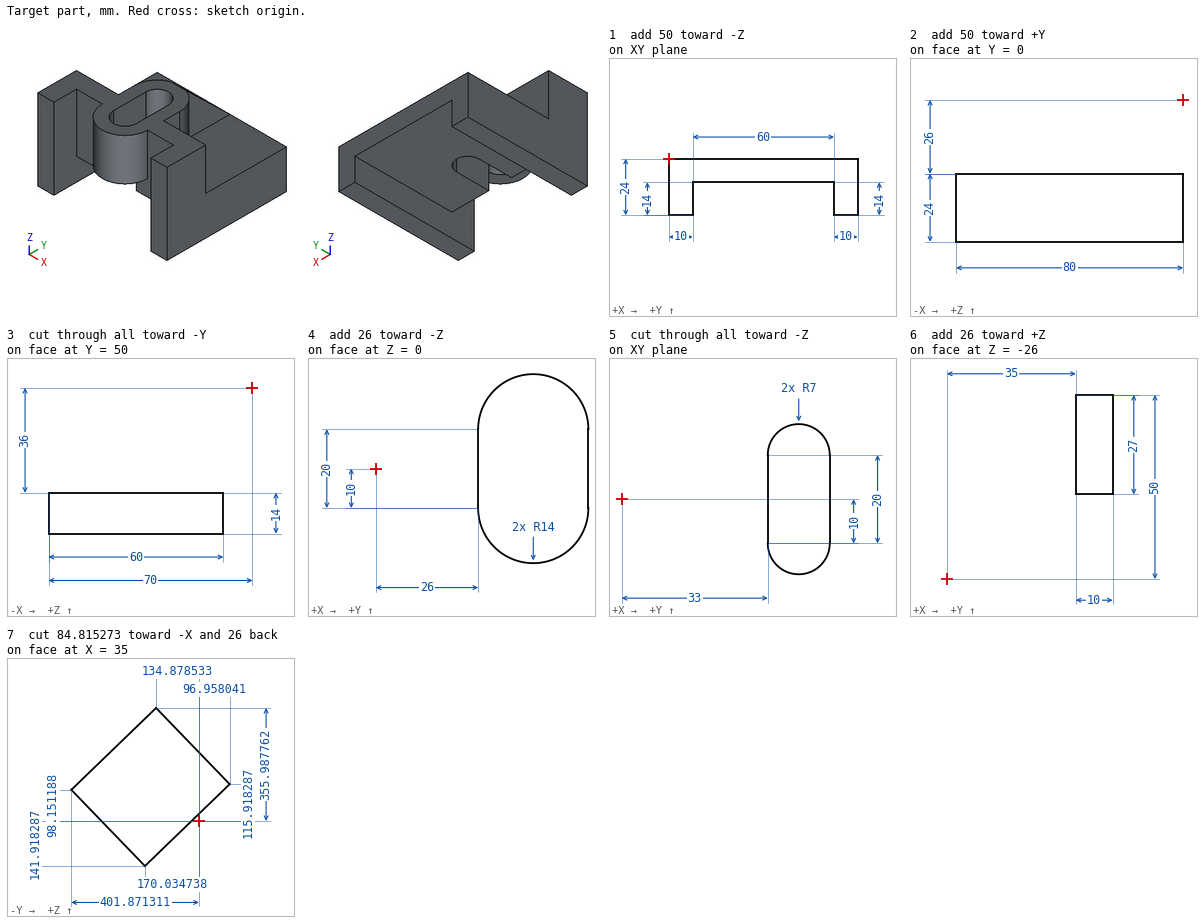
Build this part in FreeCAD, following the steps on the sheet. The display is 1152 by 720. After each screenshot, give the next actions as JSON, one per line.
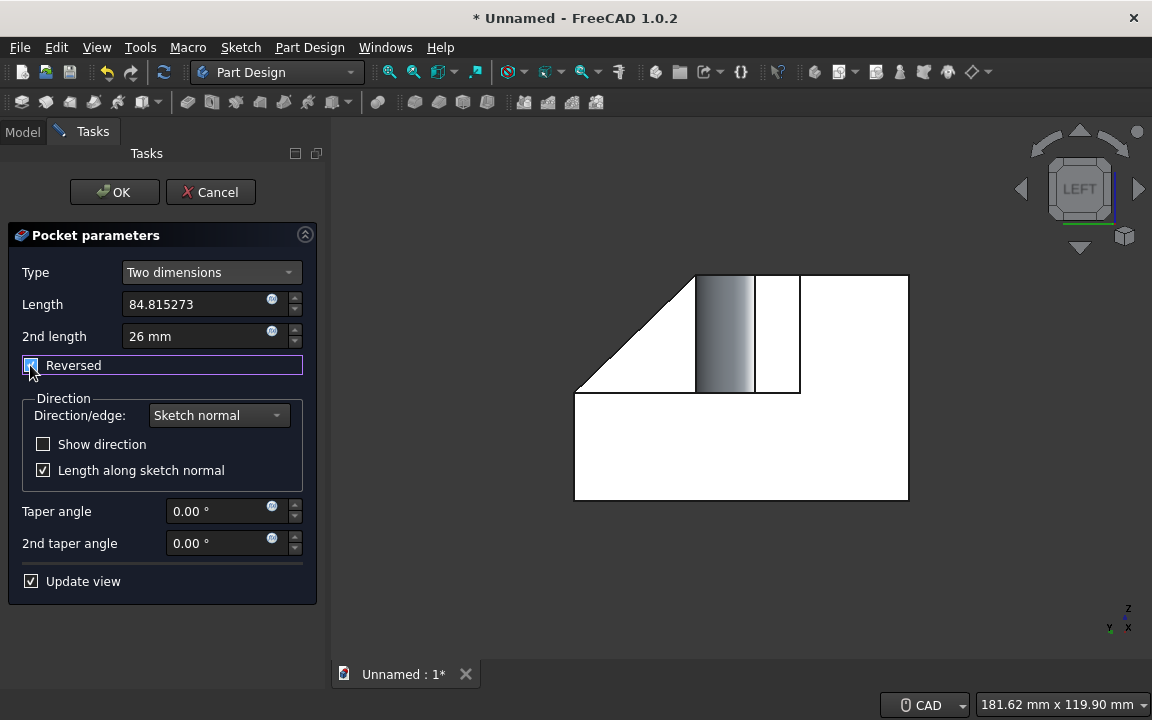
{"action": "left_click", "coordinate": [115, 192]}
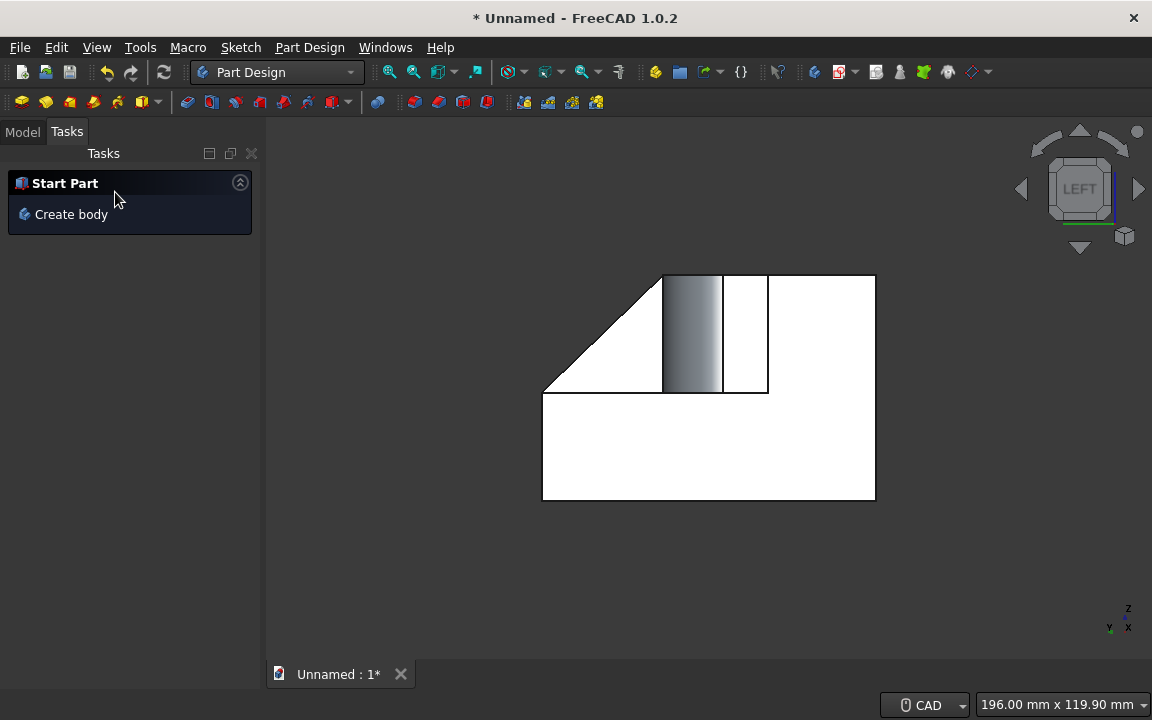
{"action": "key", "text": "0"}